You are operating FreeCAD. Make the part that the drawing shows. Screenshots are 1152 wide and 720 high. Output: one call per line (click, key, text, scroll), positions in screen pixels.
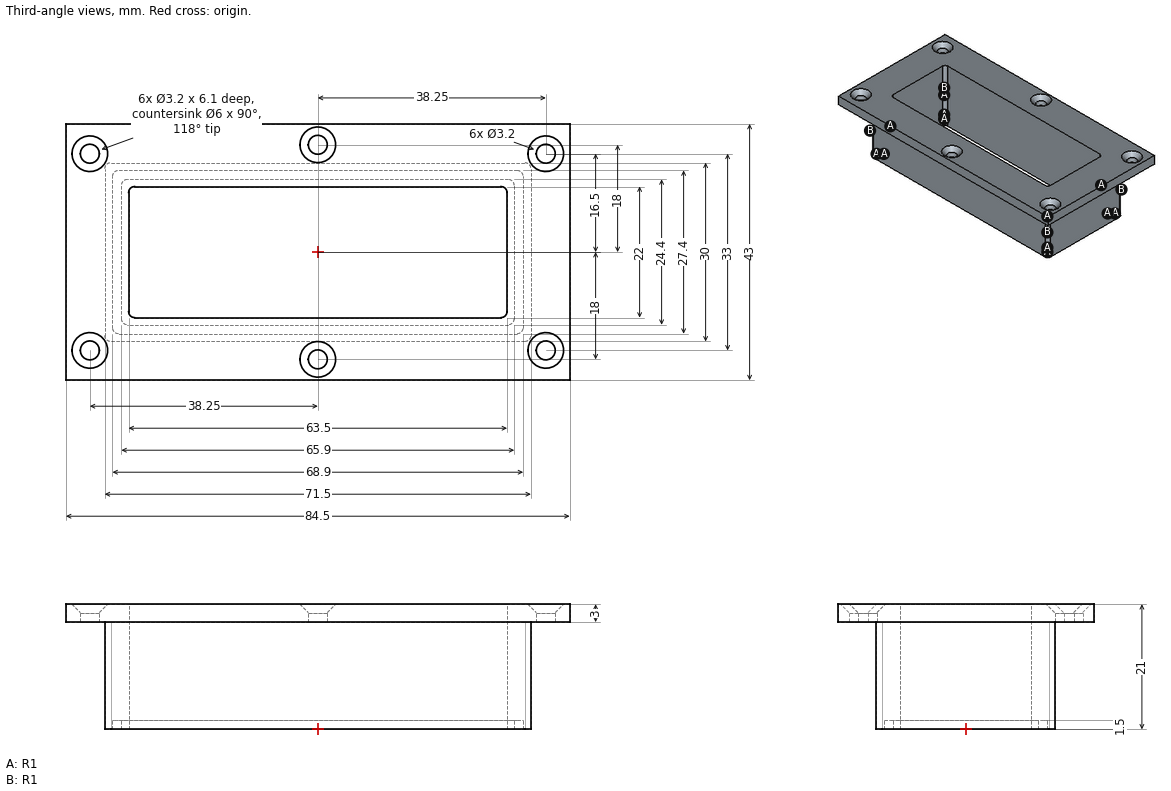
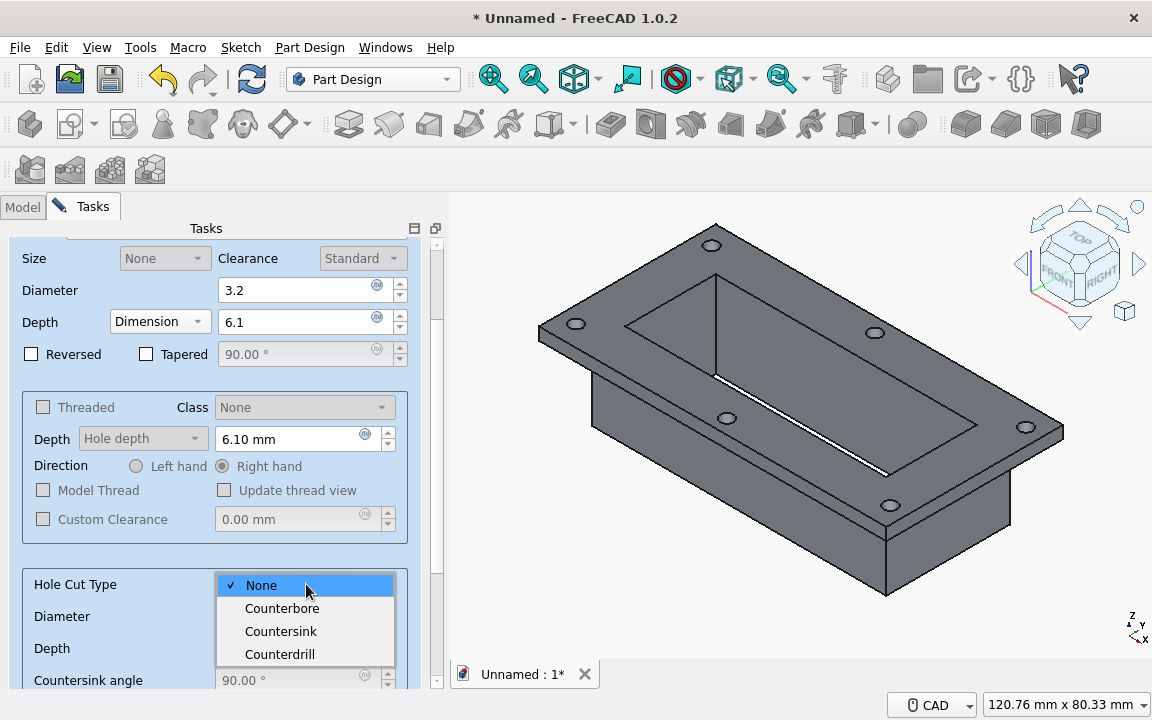
click(304, 632)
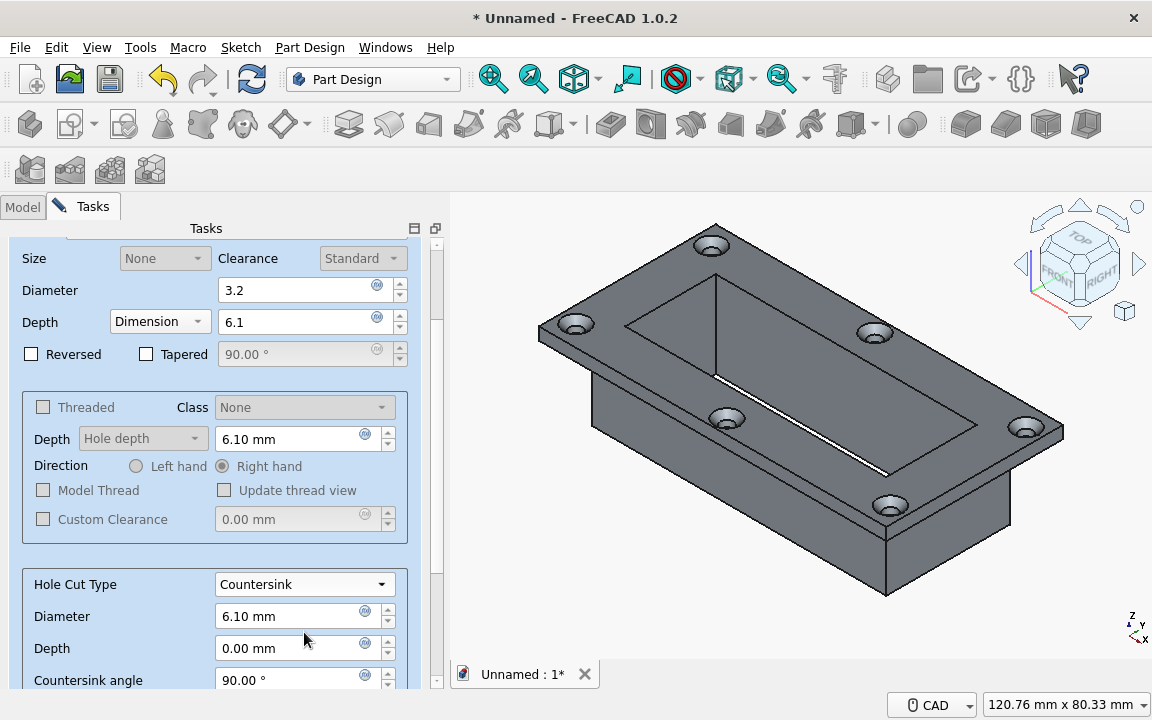
triple_click(298, 616)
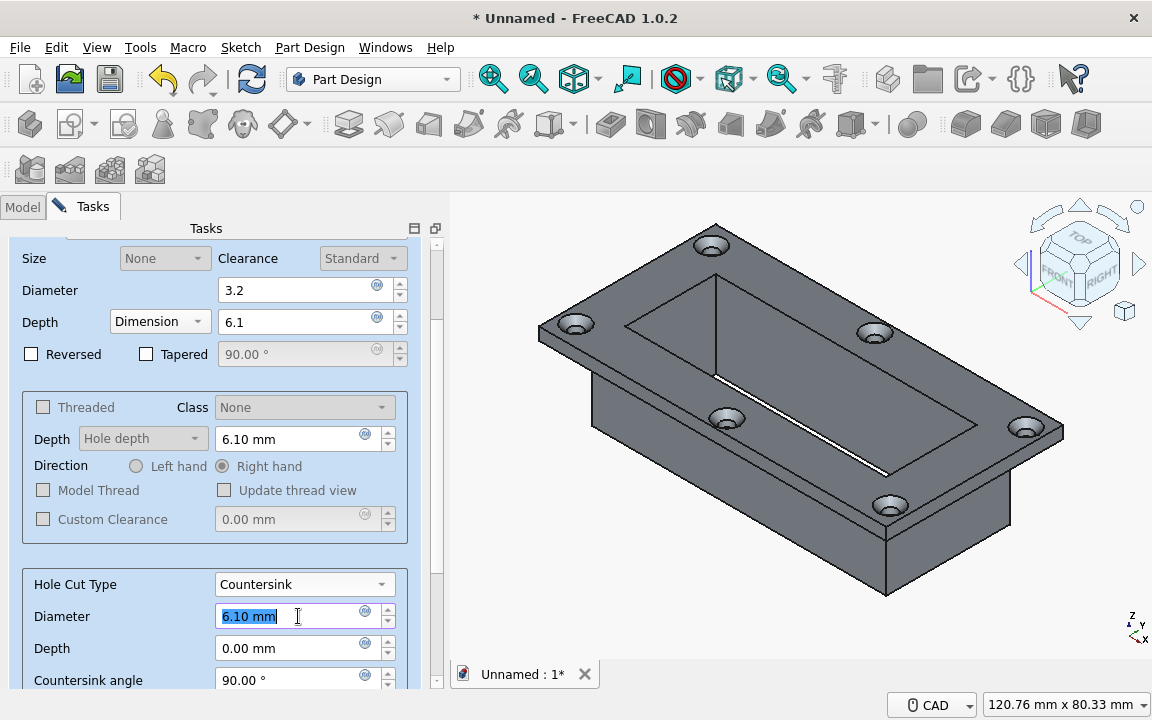
text(6)
key(Tab)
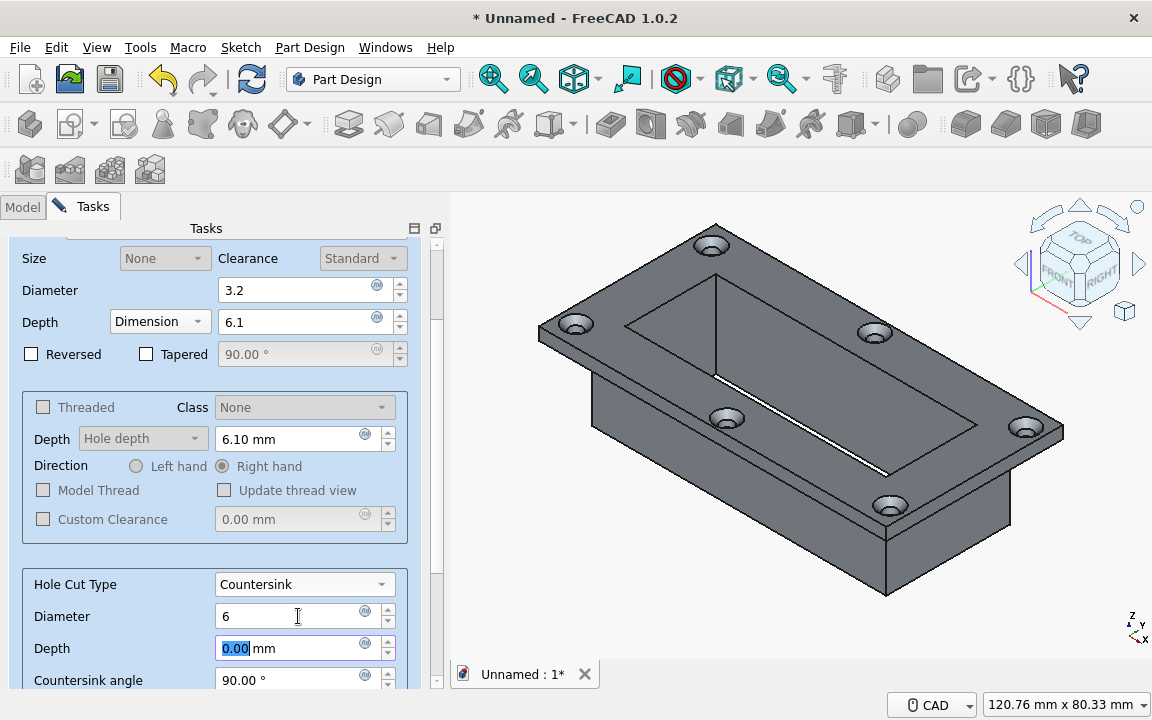
scroll(437, 463, up, 3)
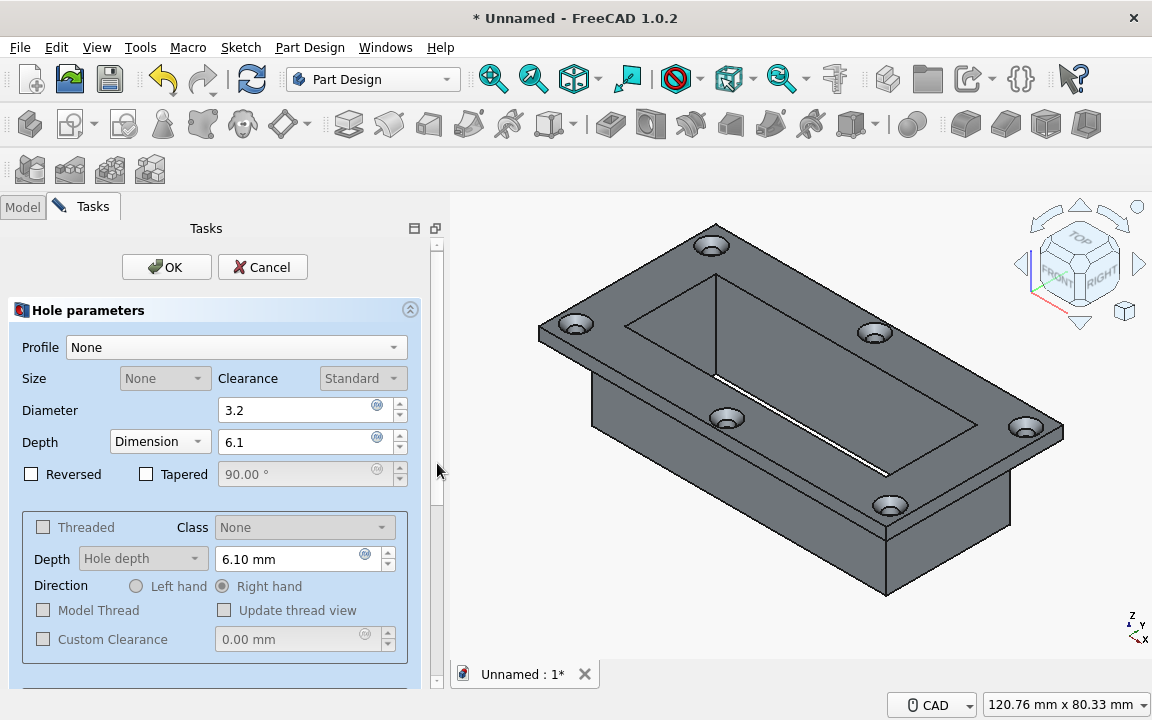
click(167, 267)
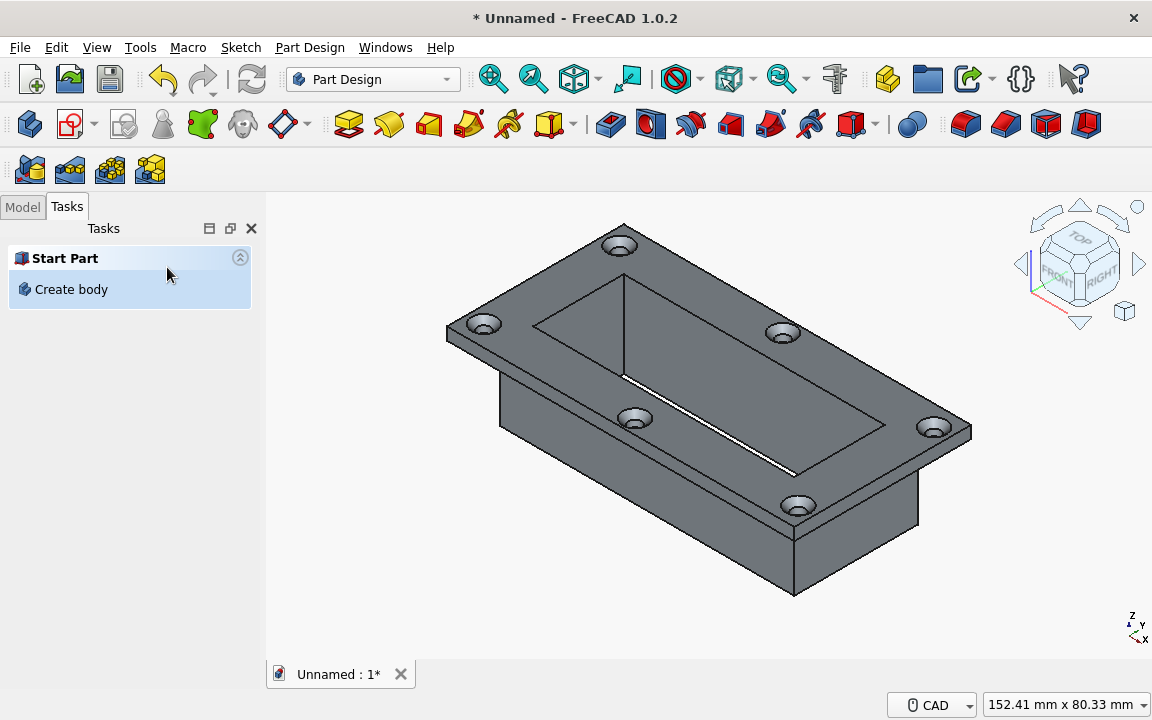
key(2)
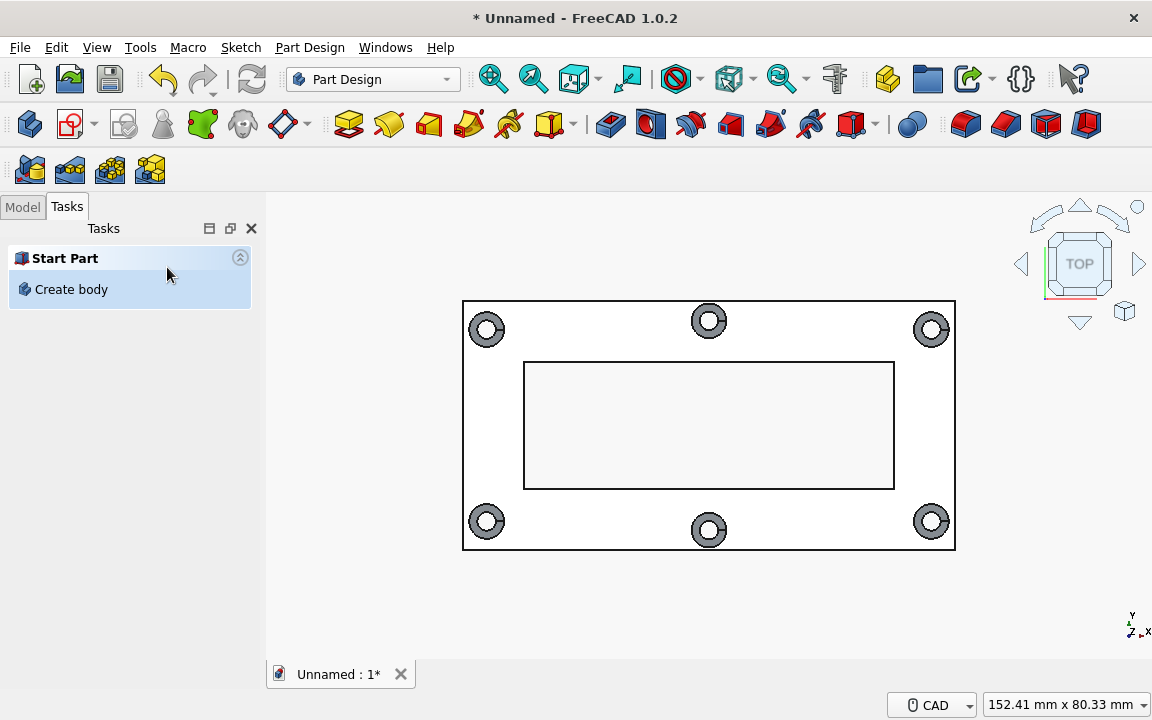
key(0)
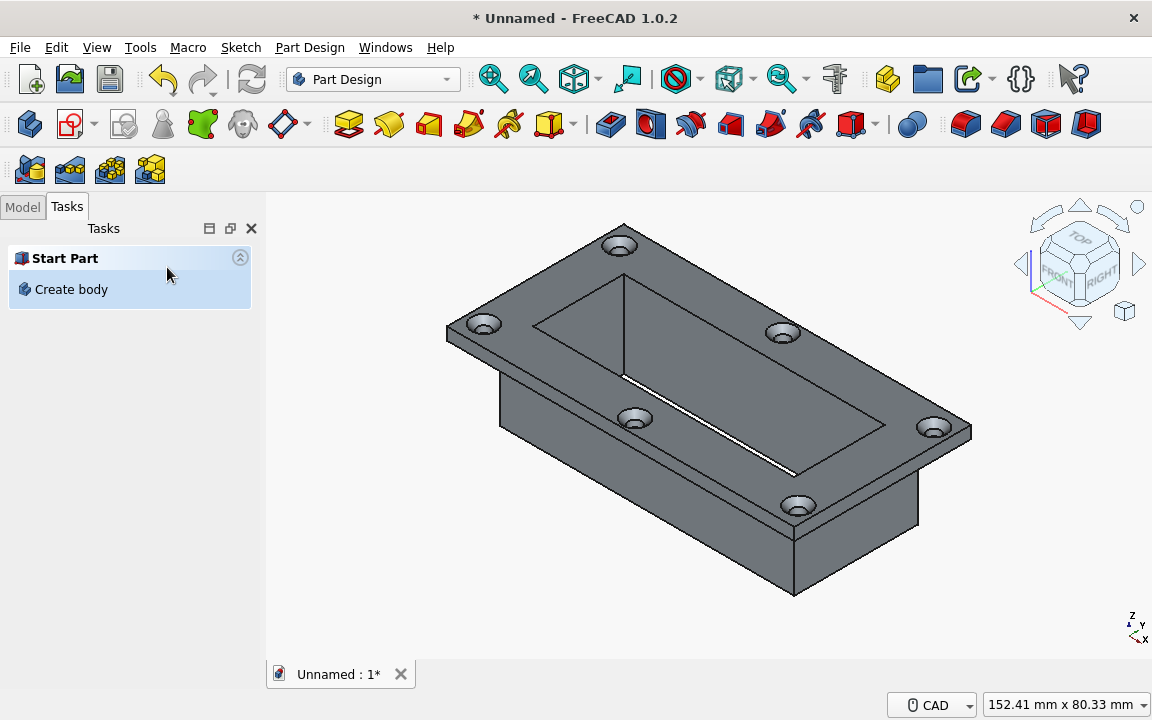
key(1)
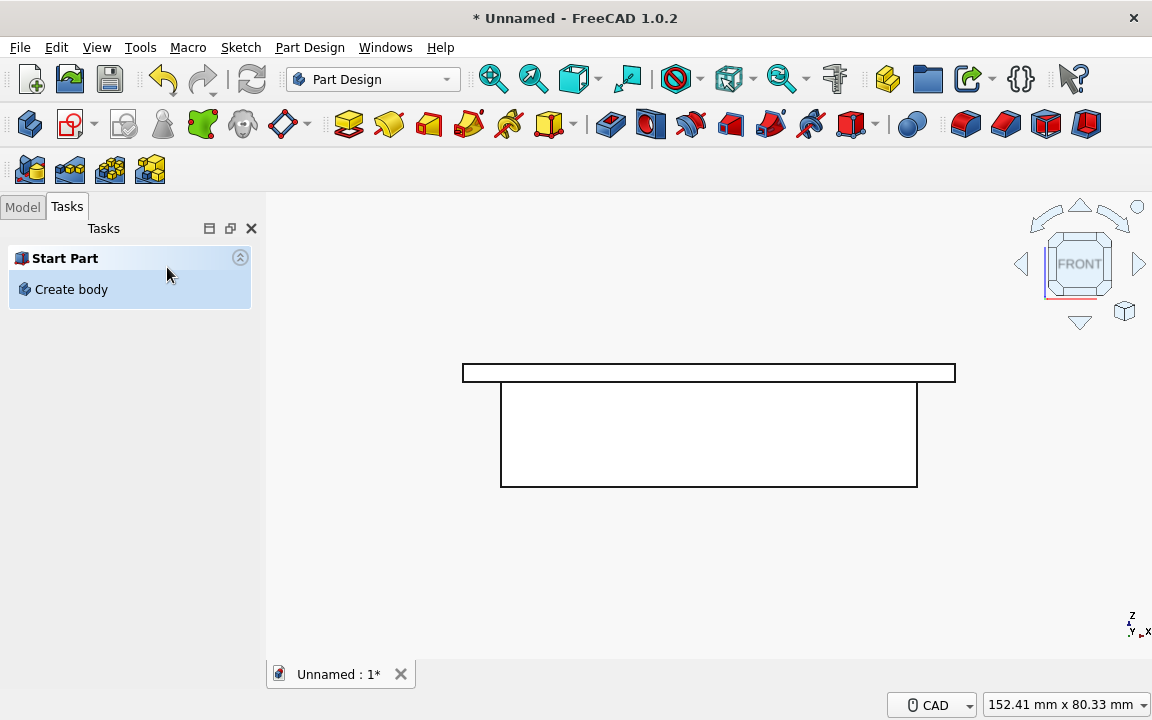
key(3)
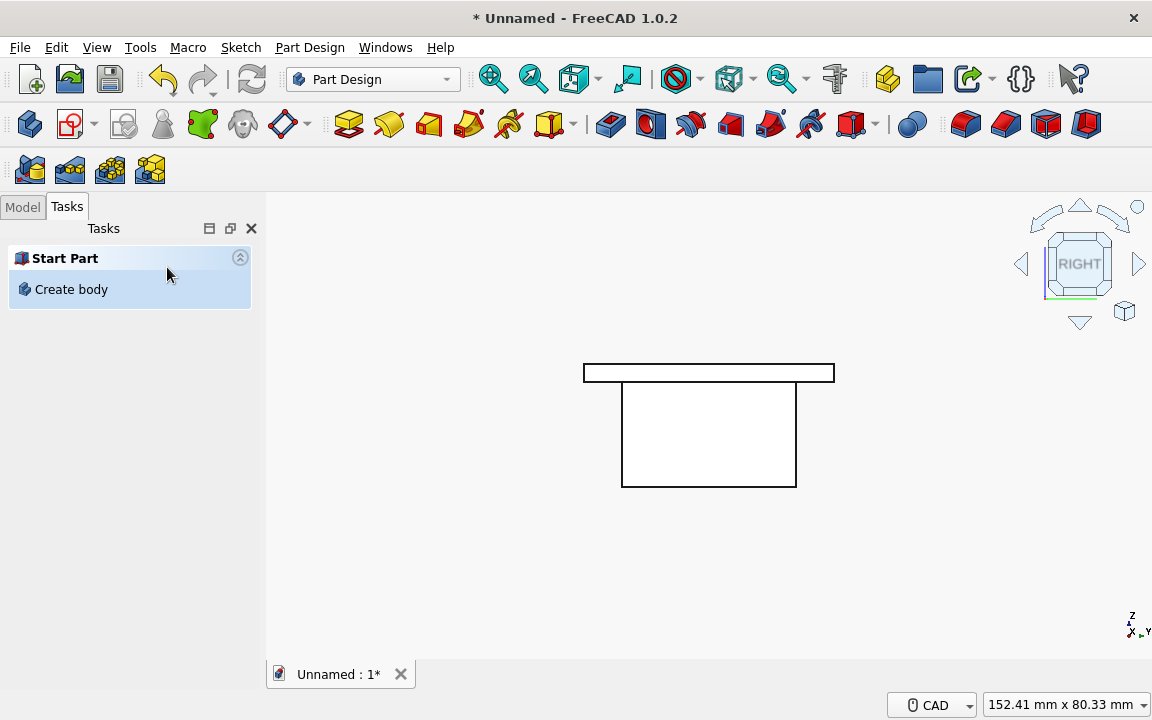
key(v)
key(f)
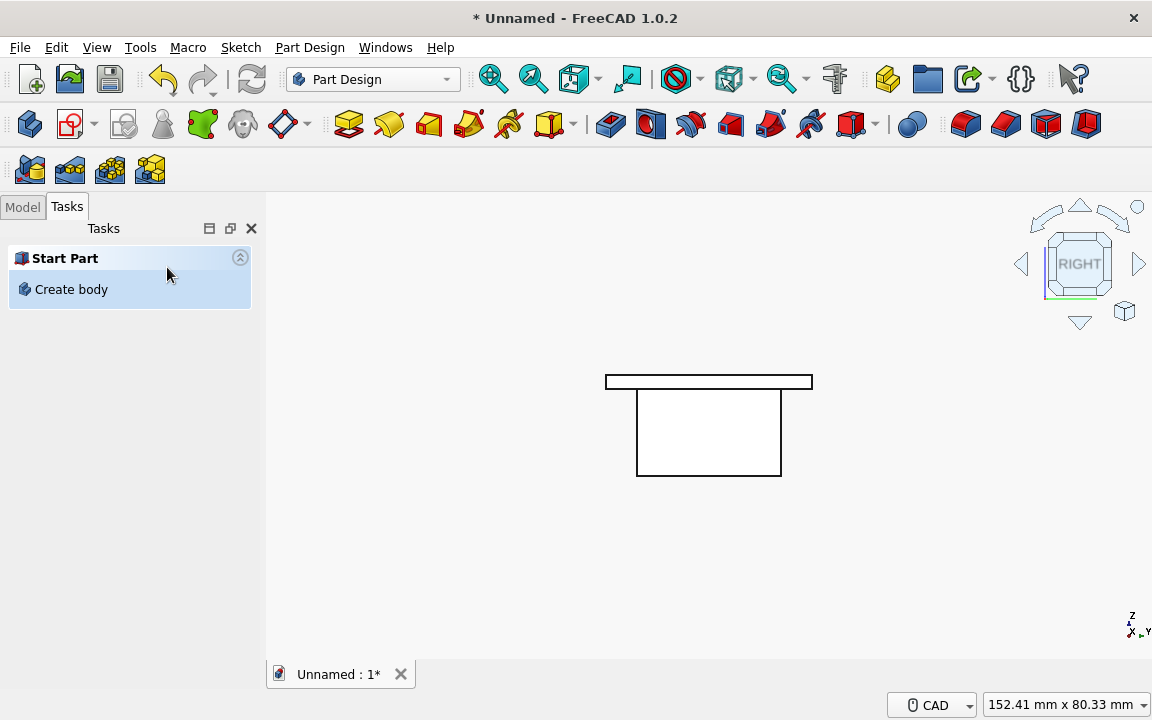
key(5)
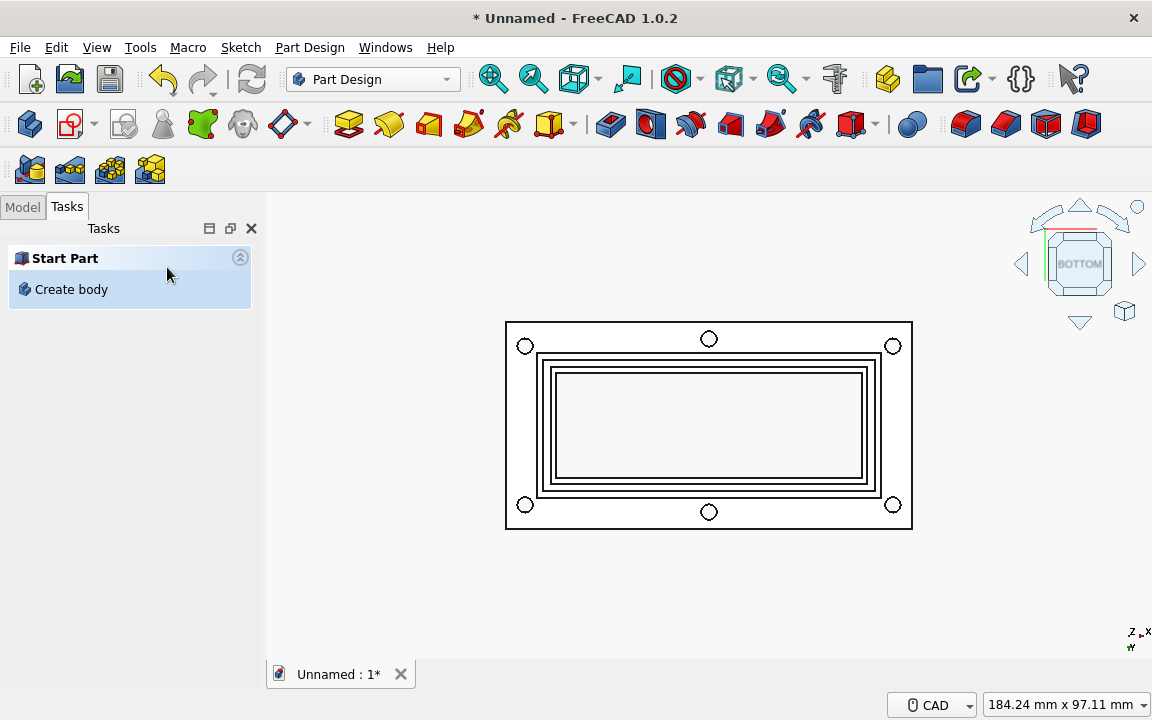
key(4)